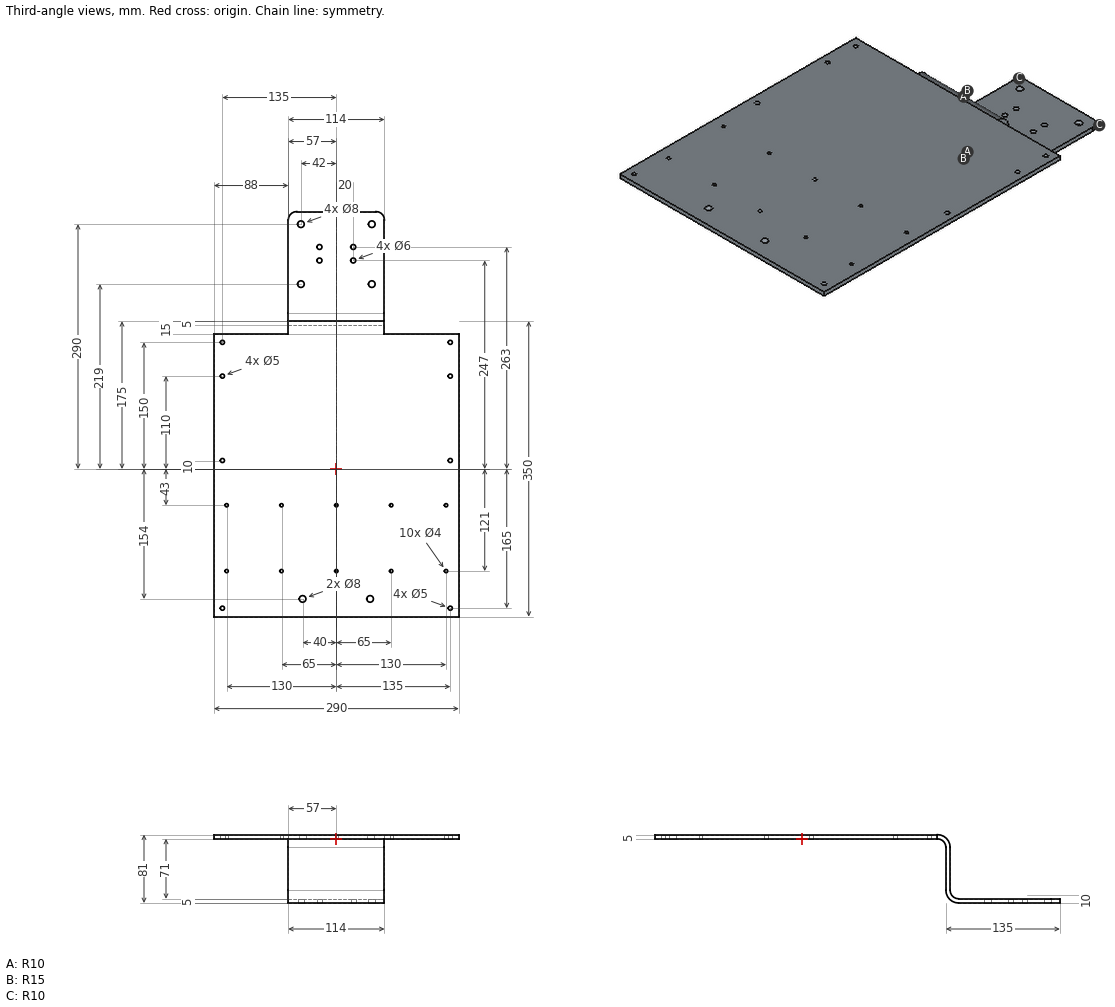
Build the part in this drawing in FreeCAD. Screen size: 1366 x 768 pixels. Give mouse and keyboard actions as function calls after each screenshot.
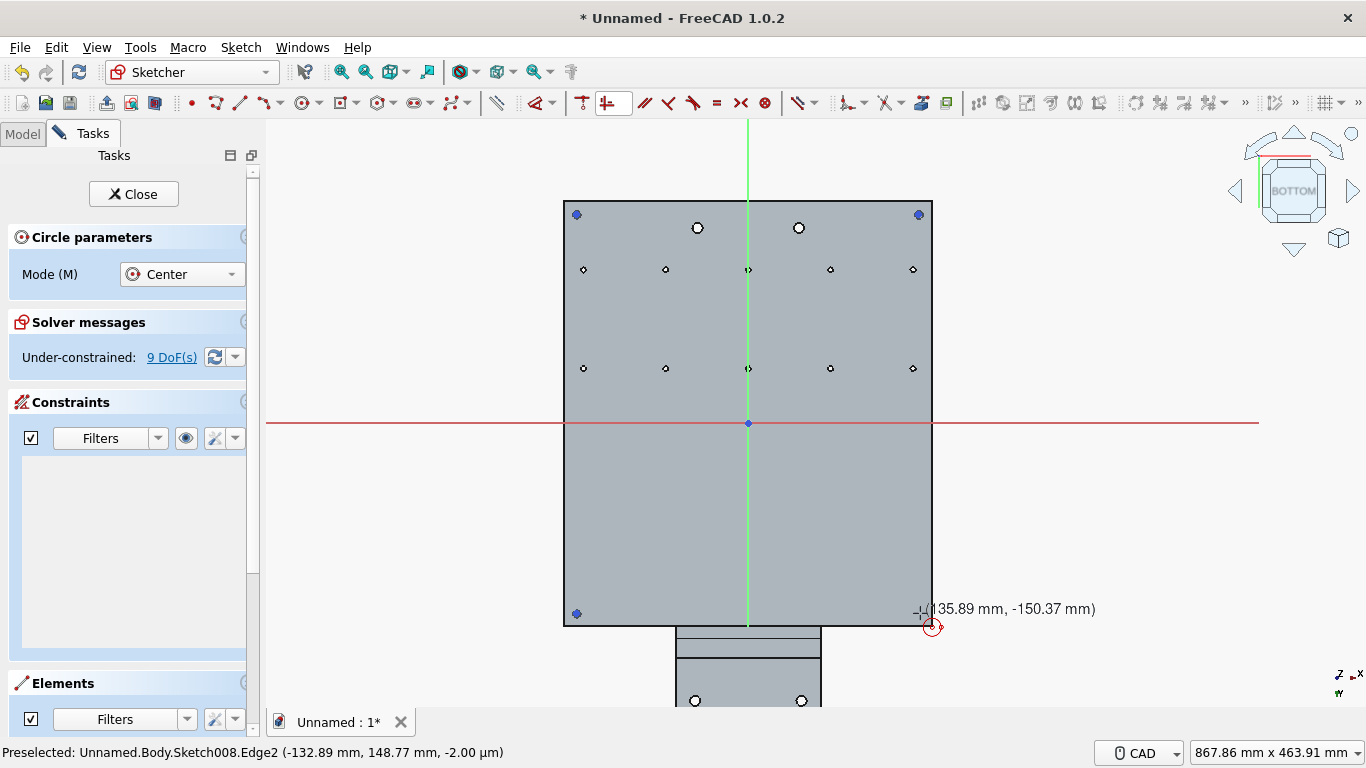
click(919, 613)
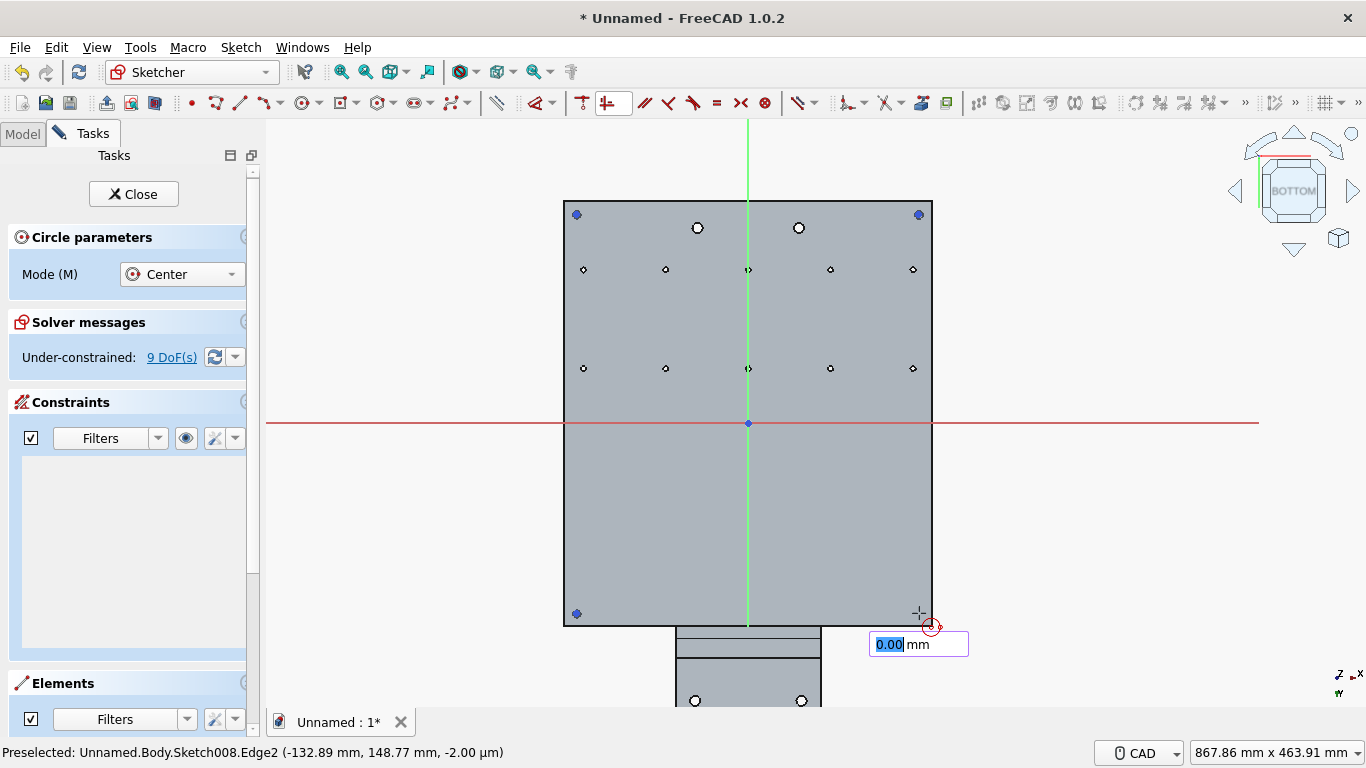
scroll(922, 611, up, 9)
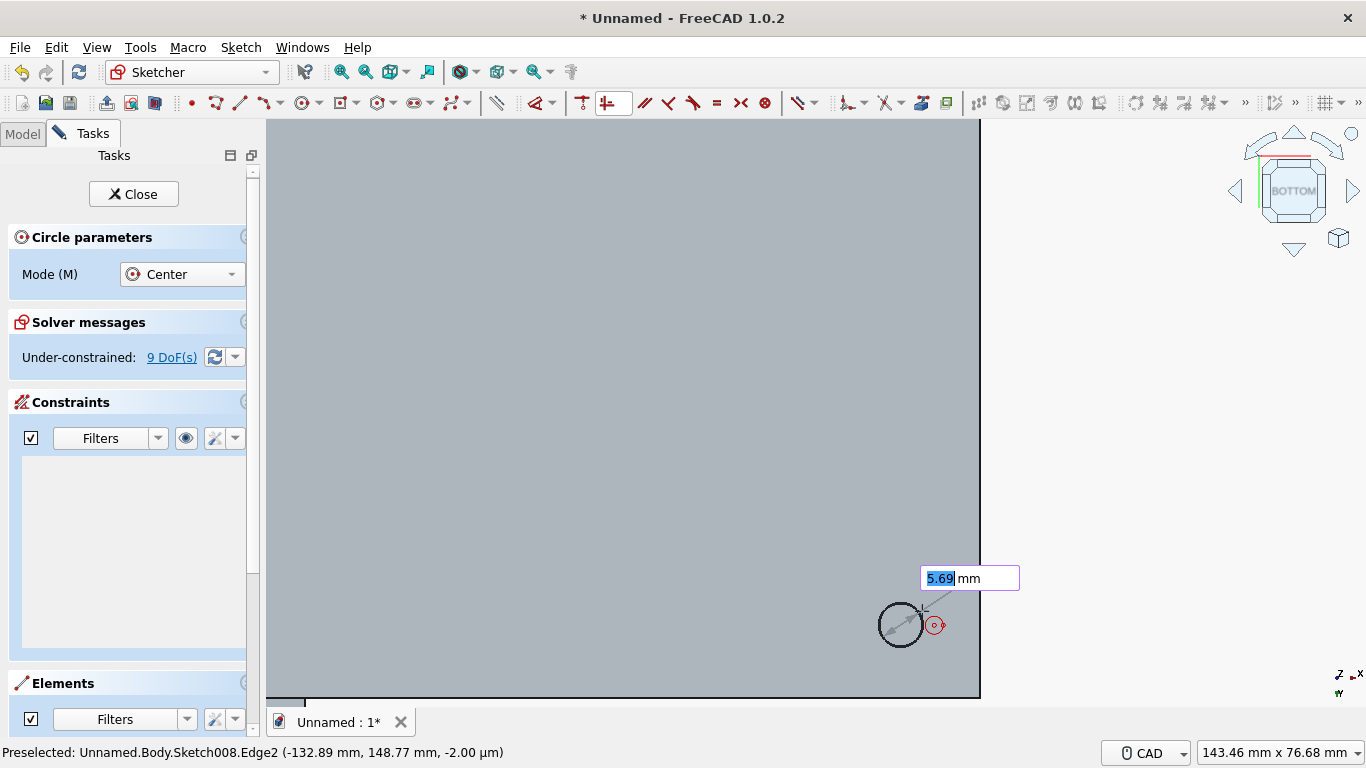
click(917, 608)
key(Escape)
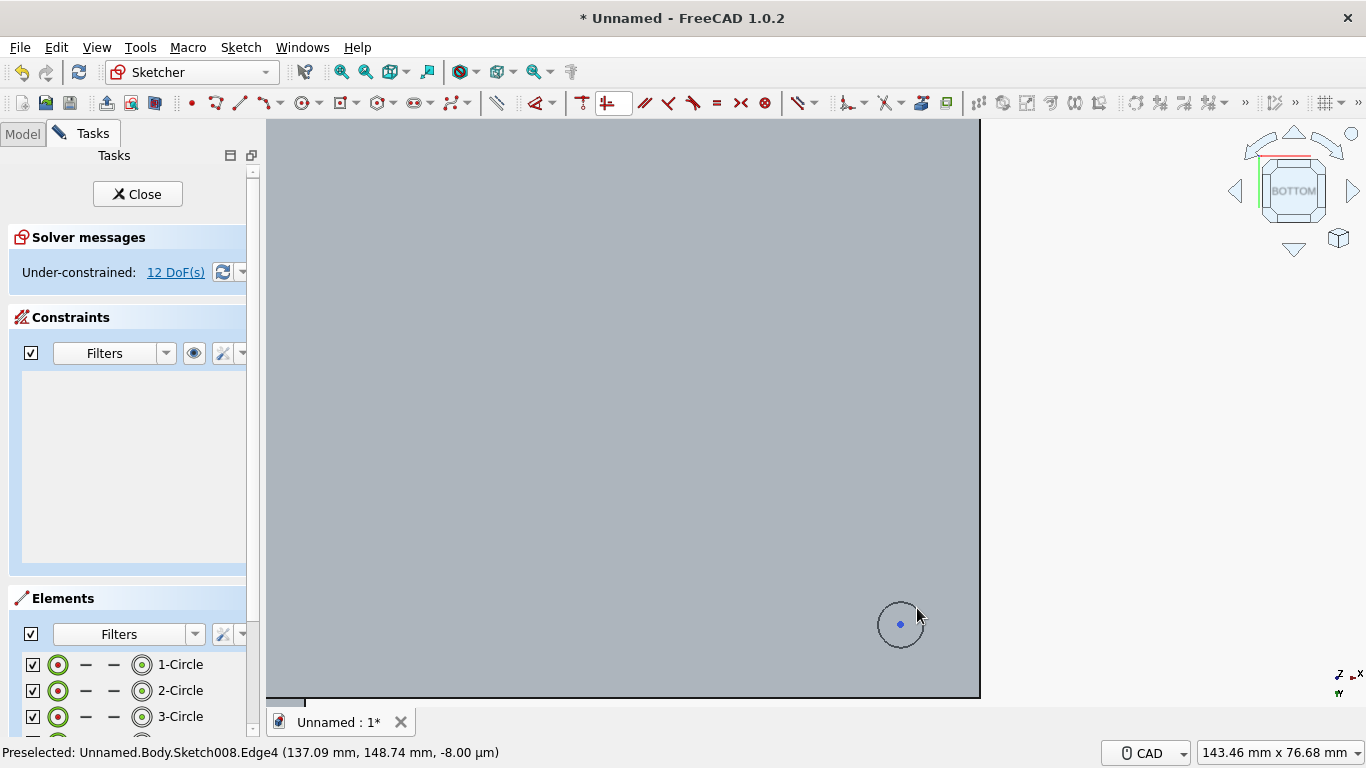
scroll(922, 611, down, 9)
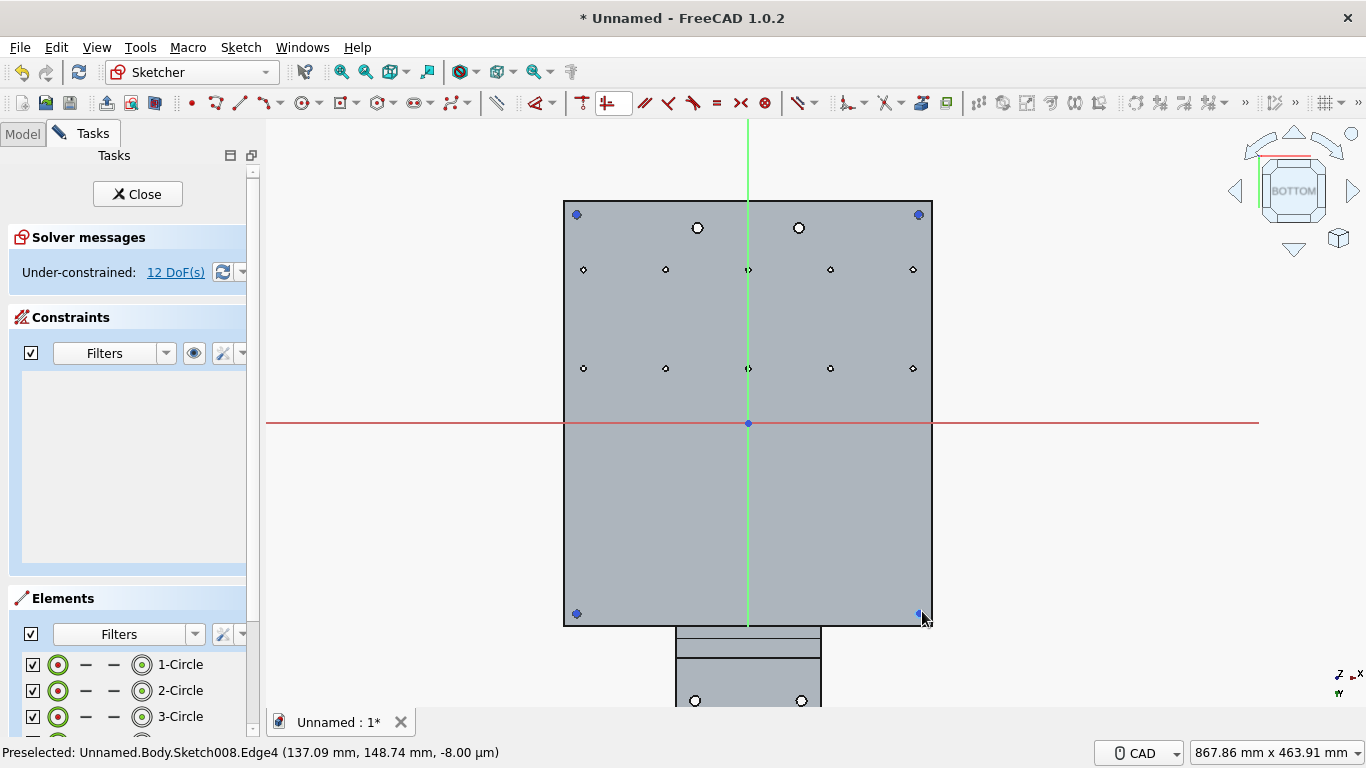
scroll(922, 212, up, 7)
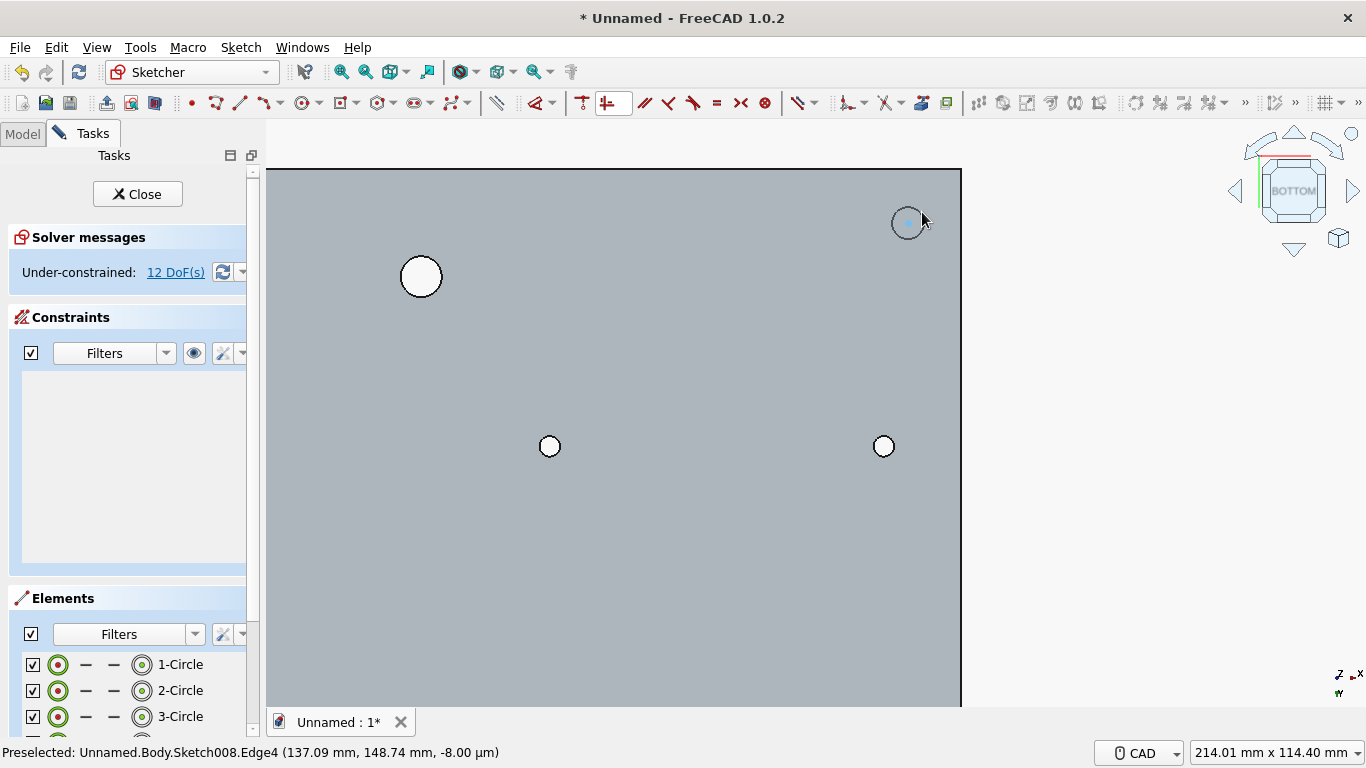
click(919, 212)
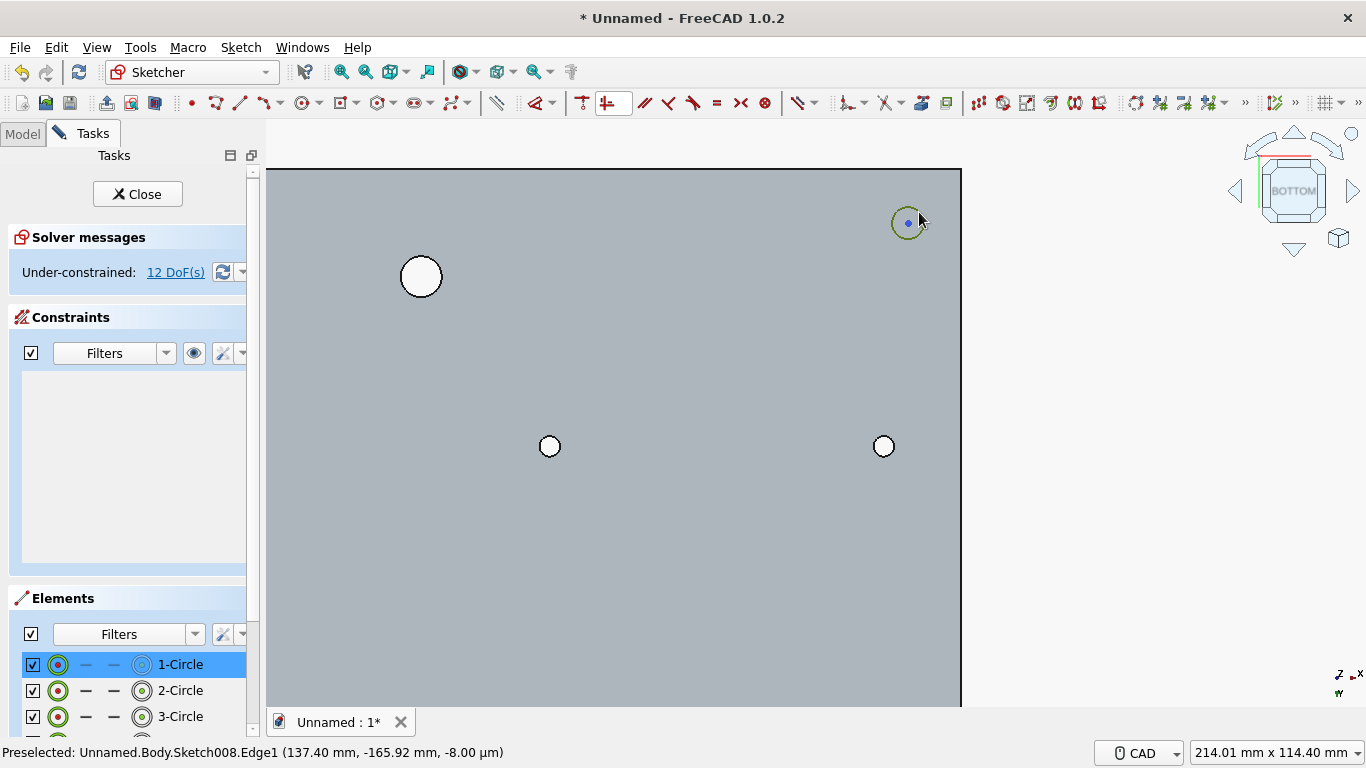
scroll(922, 211, down, 7)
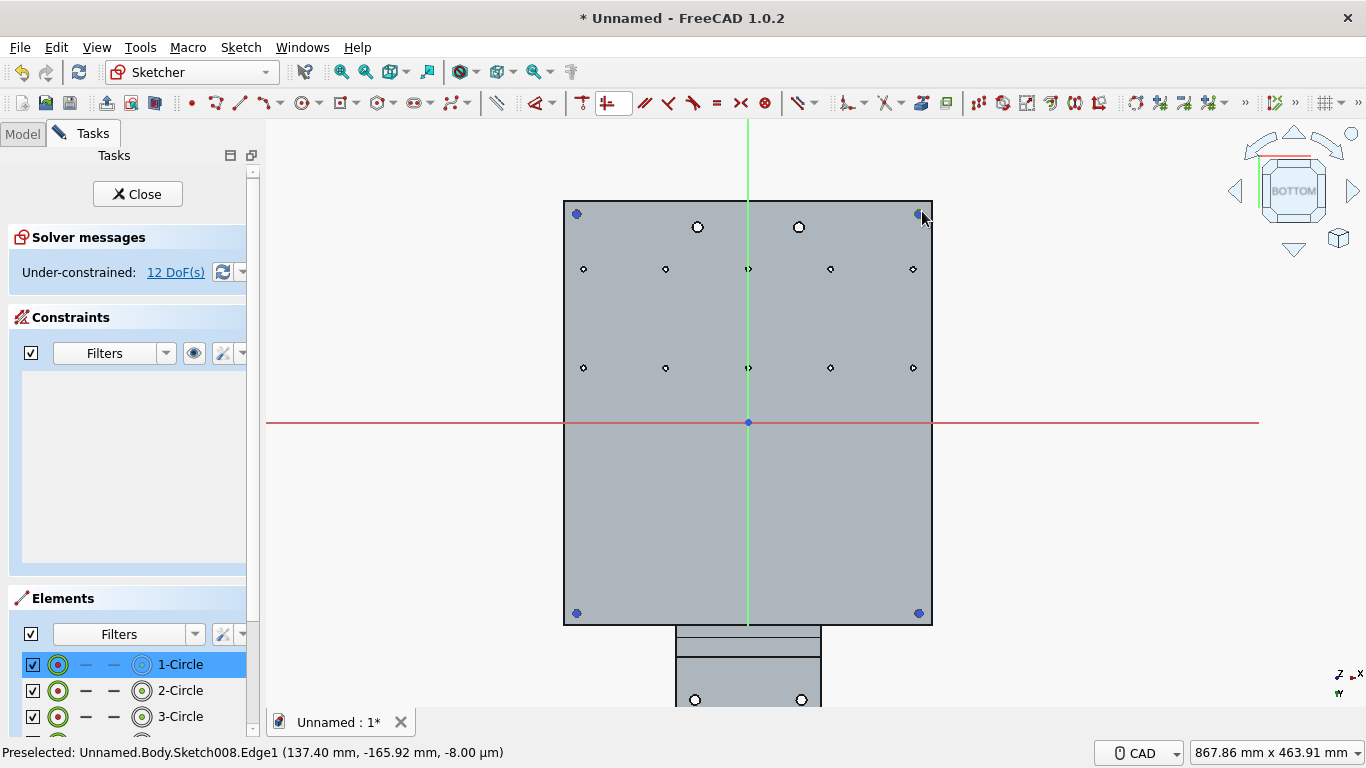
scroll(580, 211, up, 7)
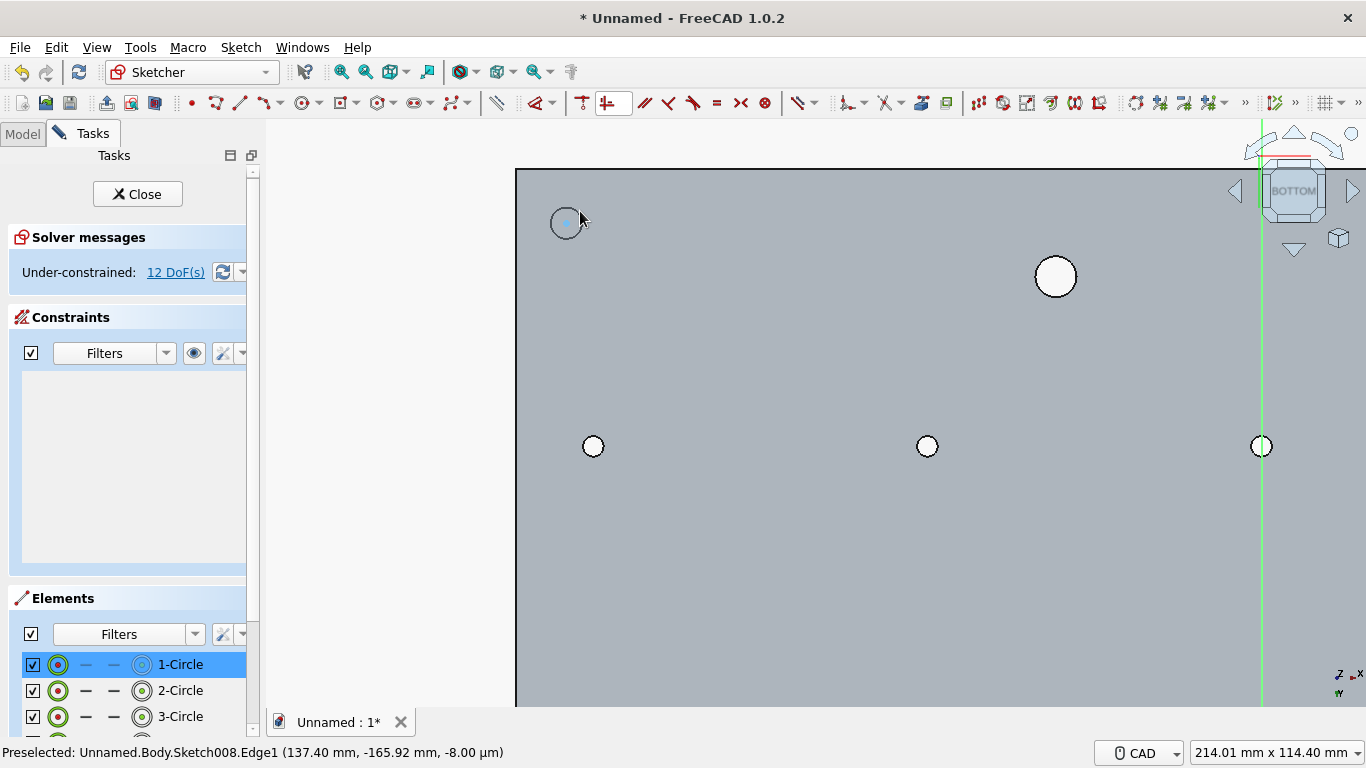
click(577, 212)